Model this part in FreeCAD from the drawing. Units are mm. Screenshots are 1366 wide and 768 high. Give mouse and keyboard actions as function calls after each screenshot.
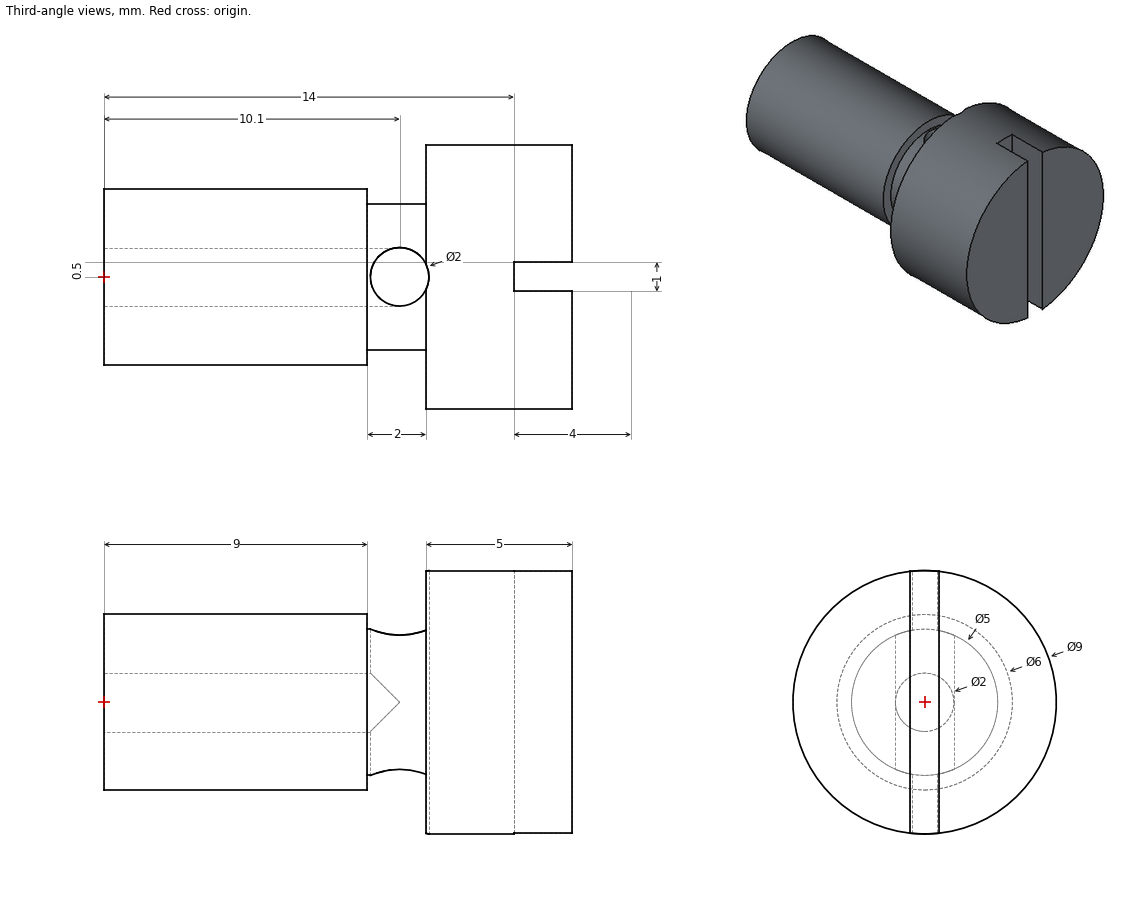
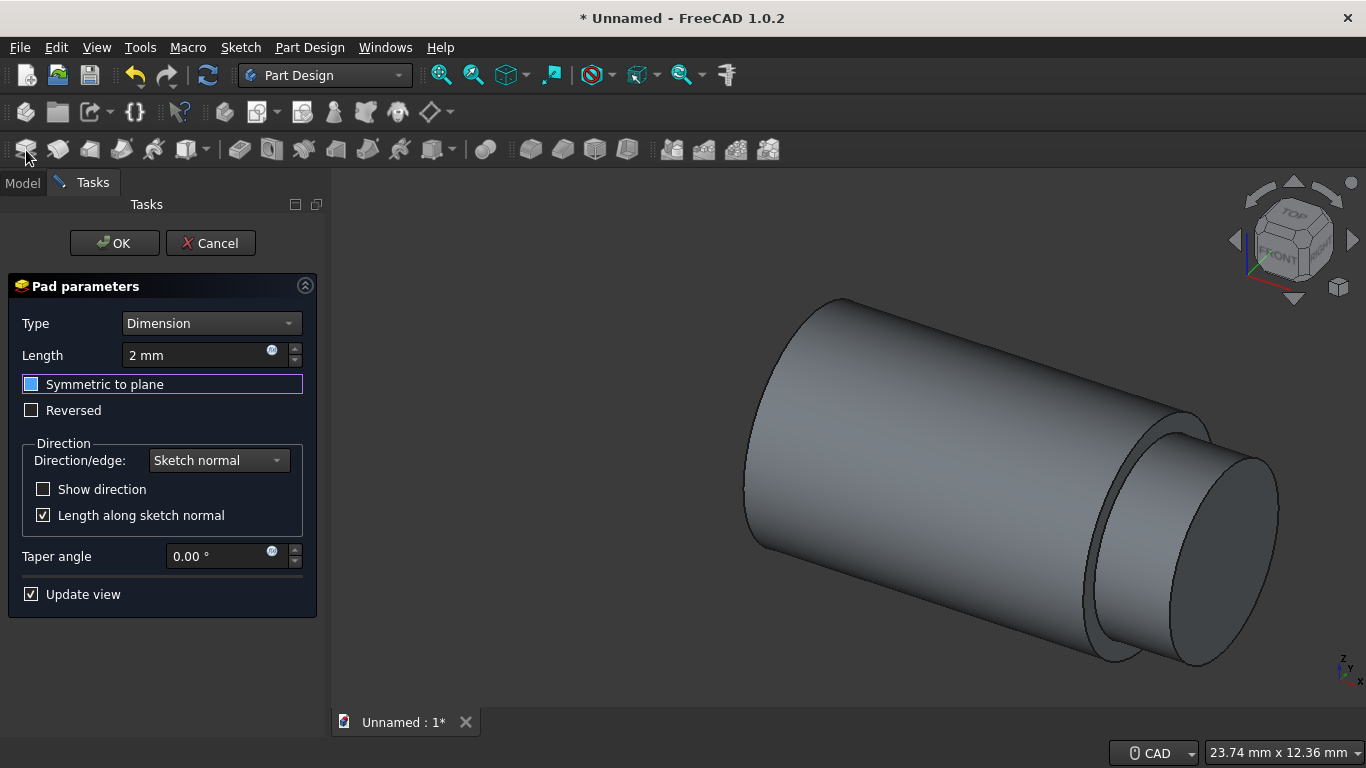
click(115, 243)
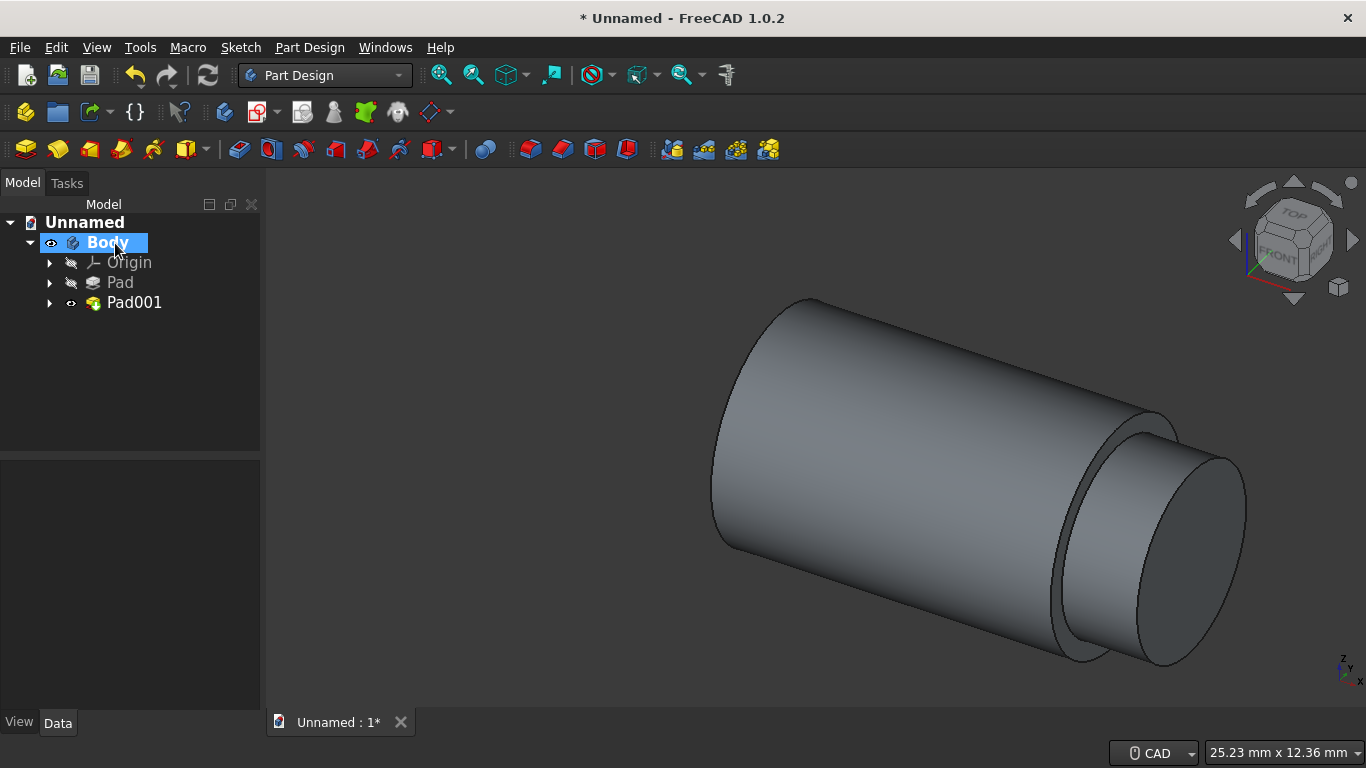
click(442, 76)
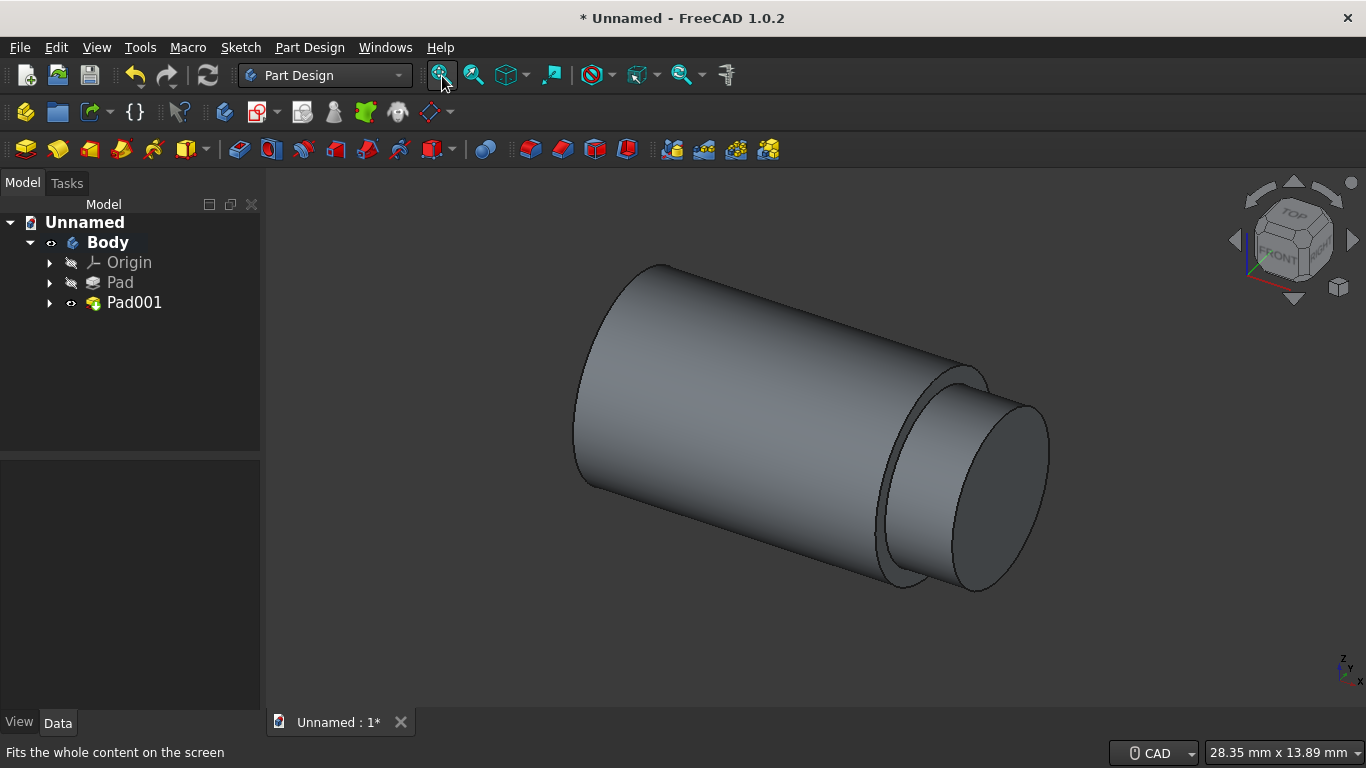
click(1001, 498)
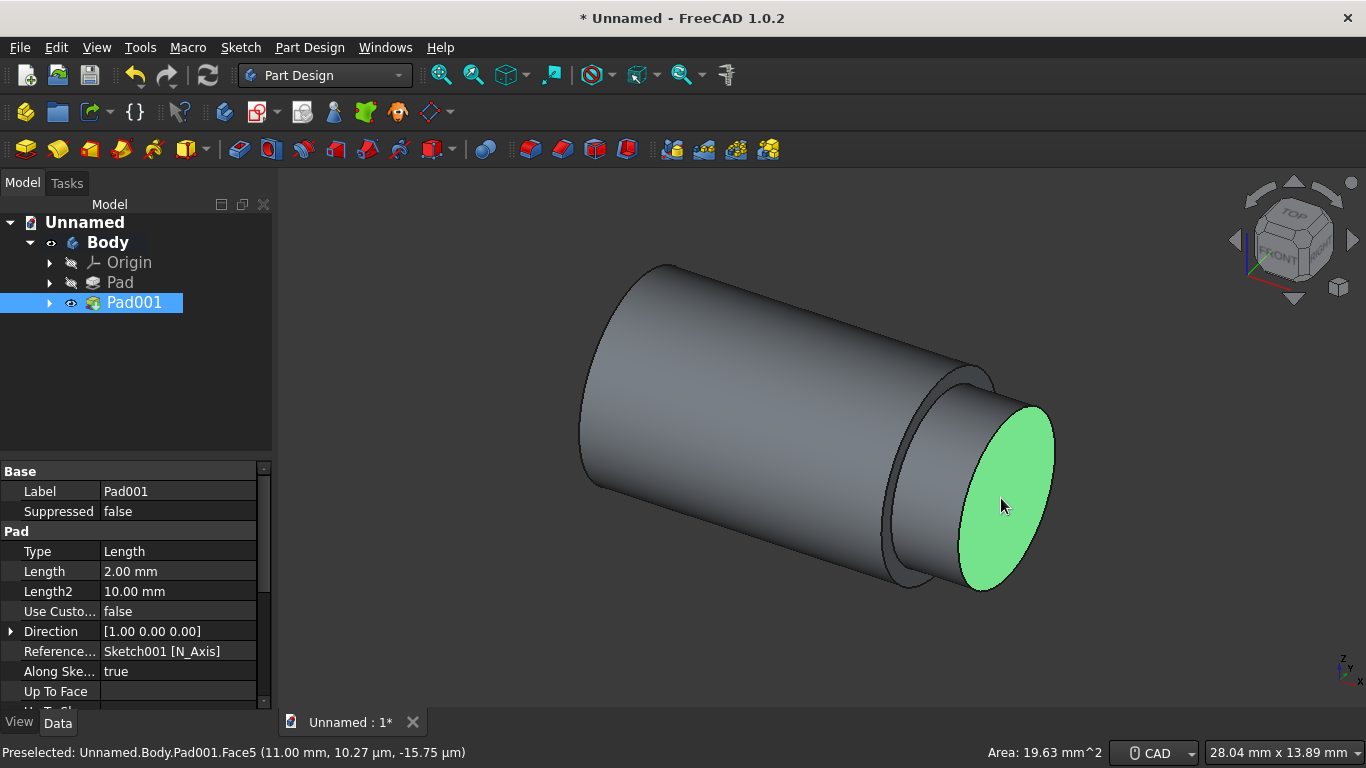
click(258, 112)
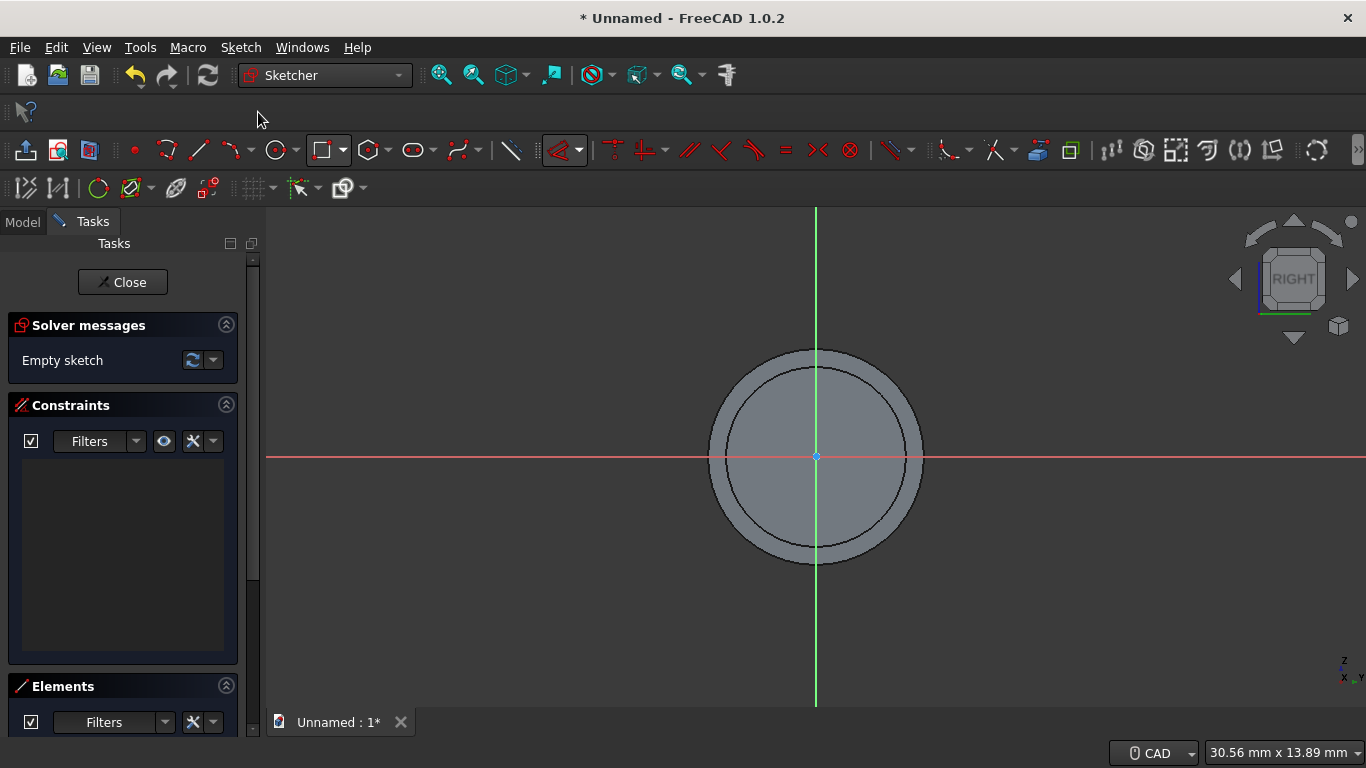
click(276, 150)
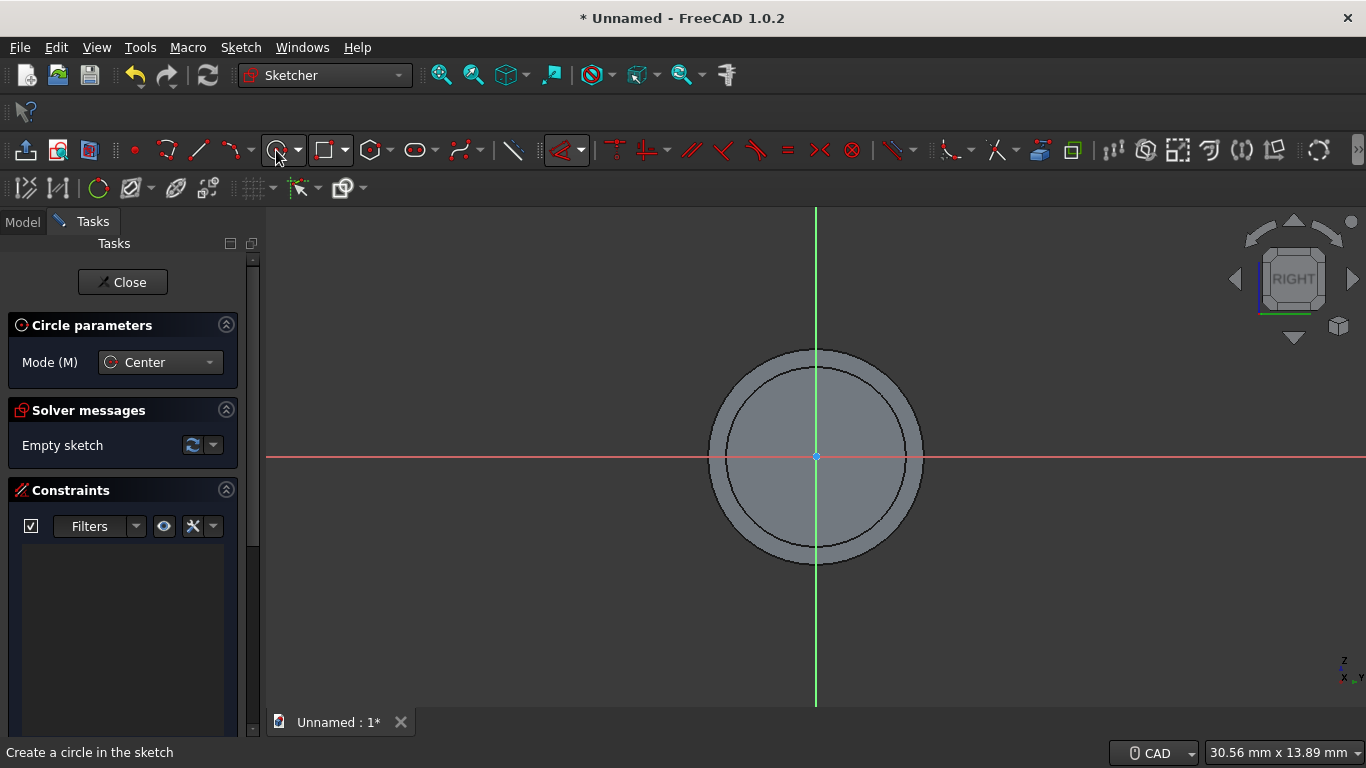
click(816, 457)
click(931, 342)
key(Escape)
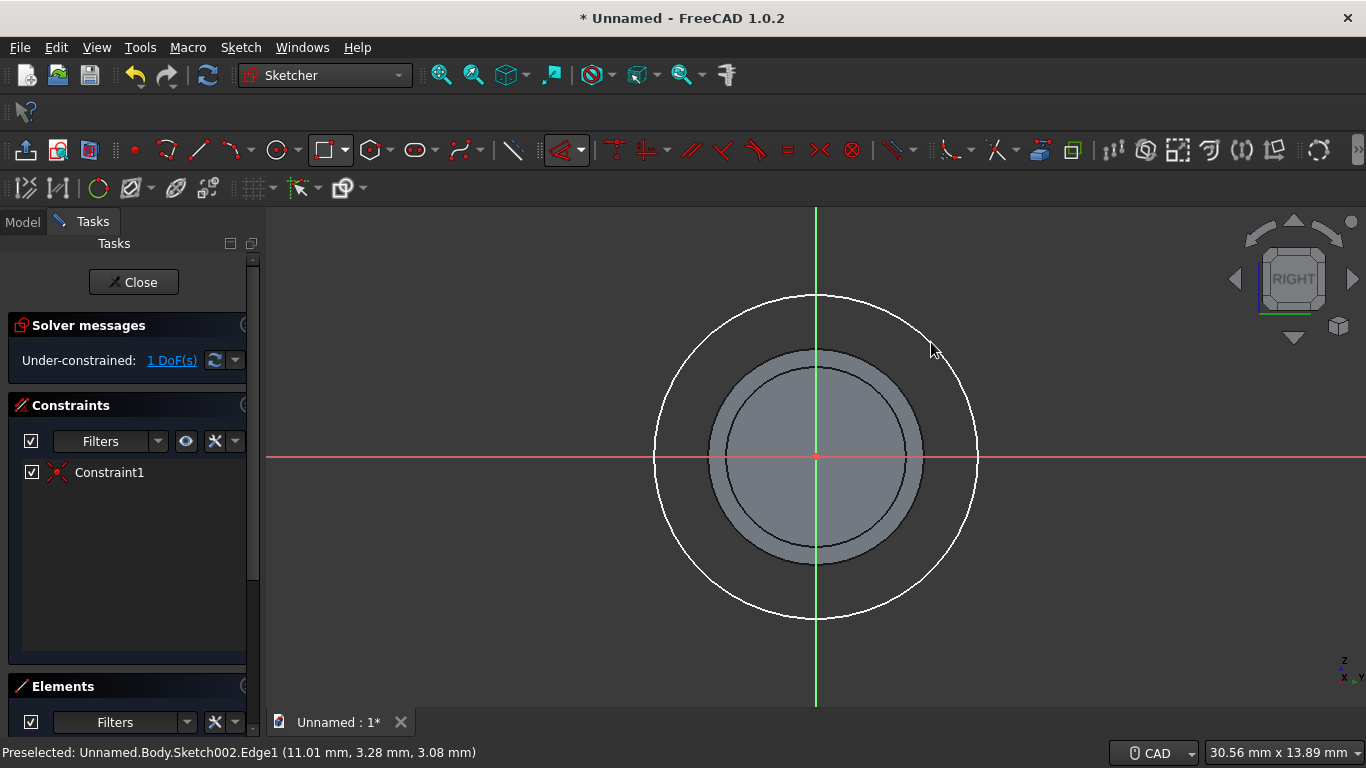
click(930, 342)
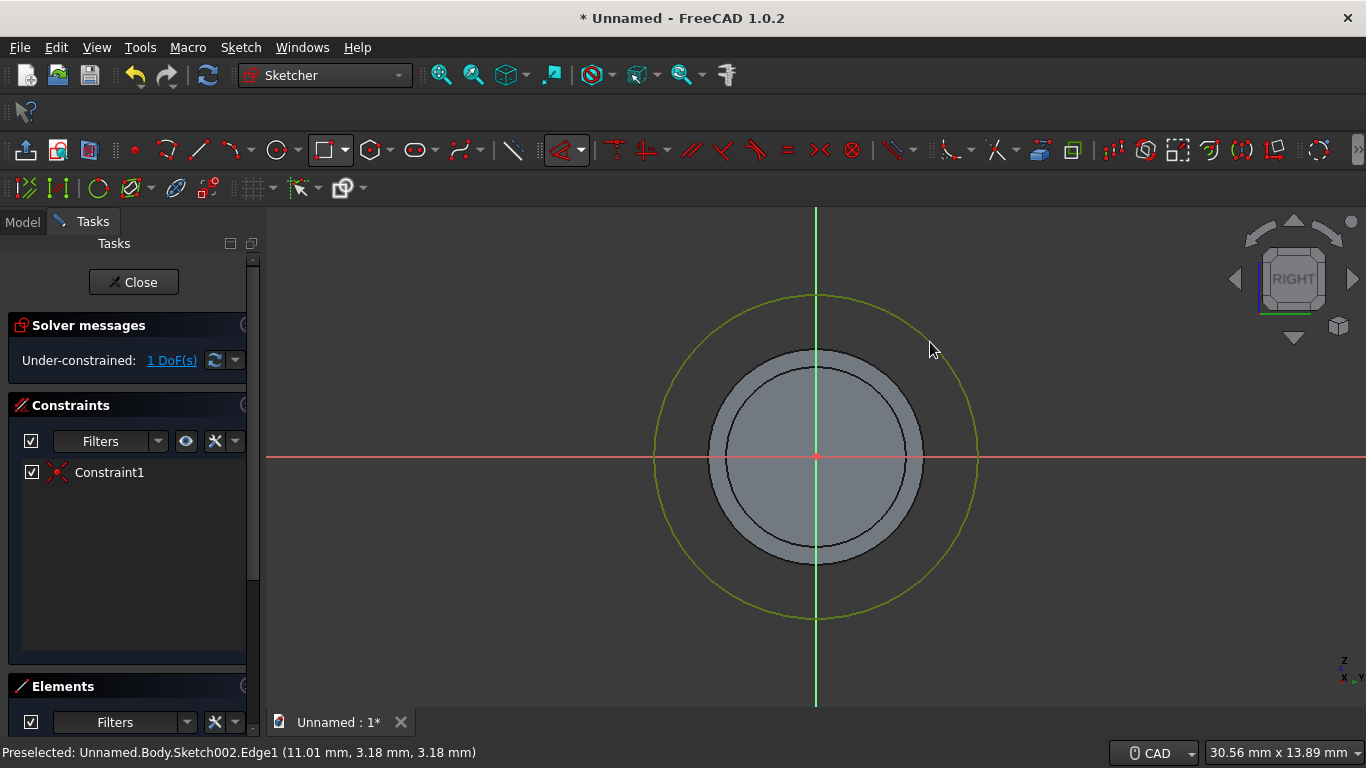
click(584, 150)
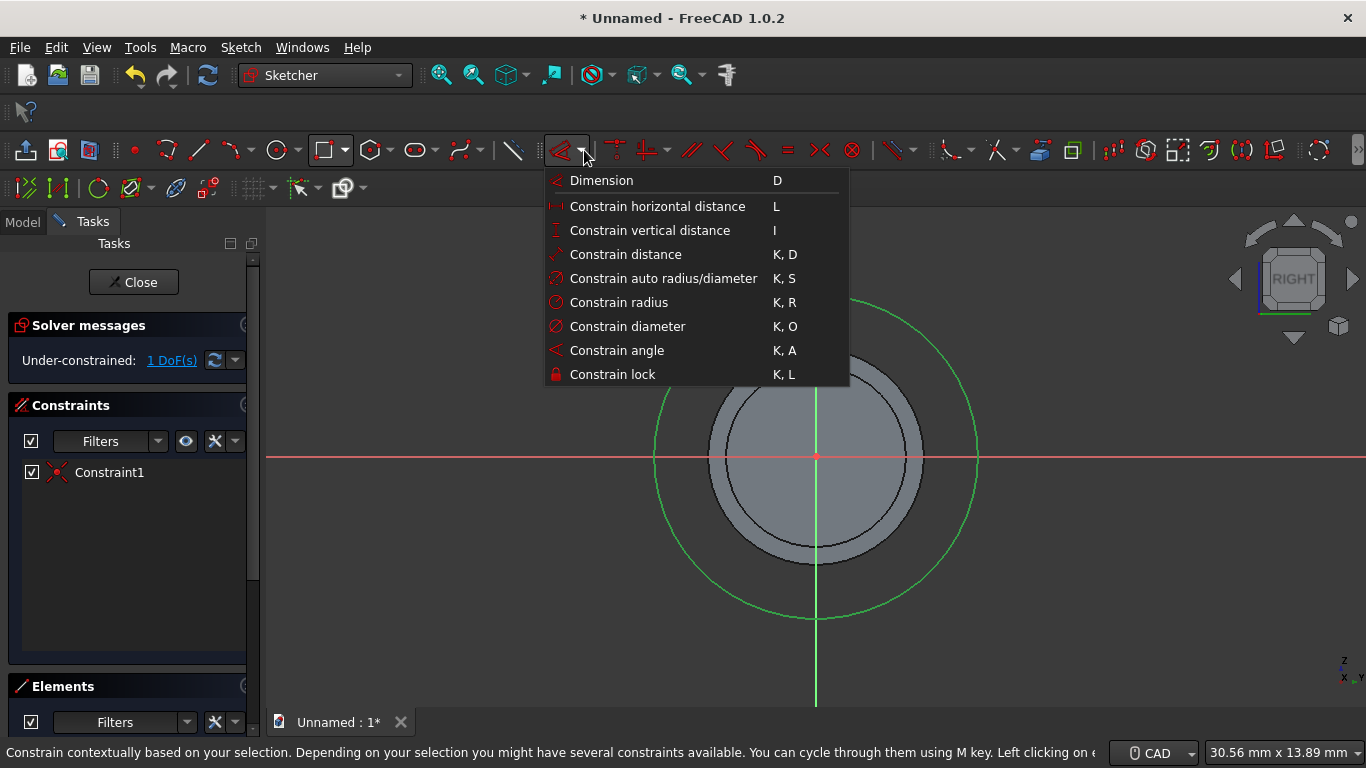
click(697, 326)